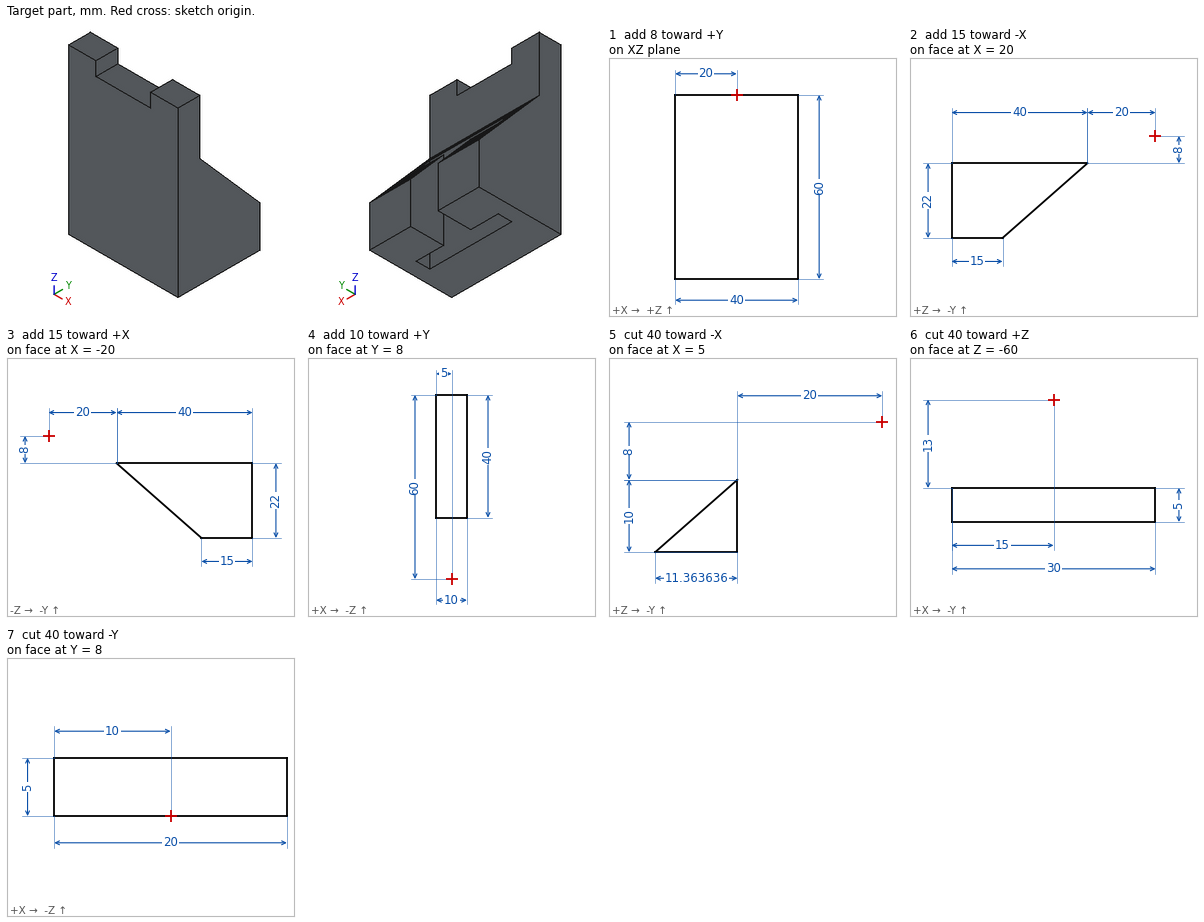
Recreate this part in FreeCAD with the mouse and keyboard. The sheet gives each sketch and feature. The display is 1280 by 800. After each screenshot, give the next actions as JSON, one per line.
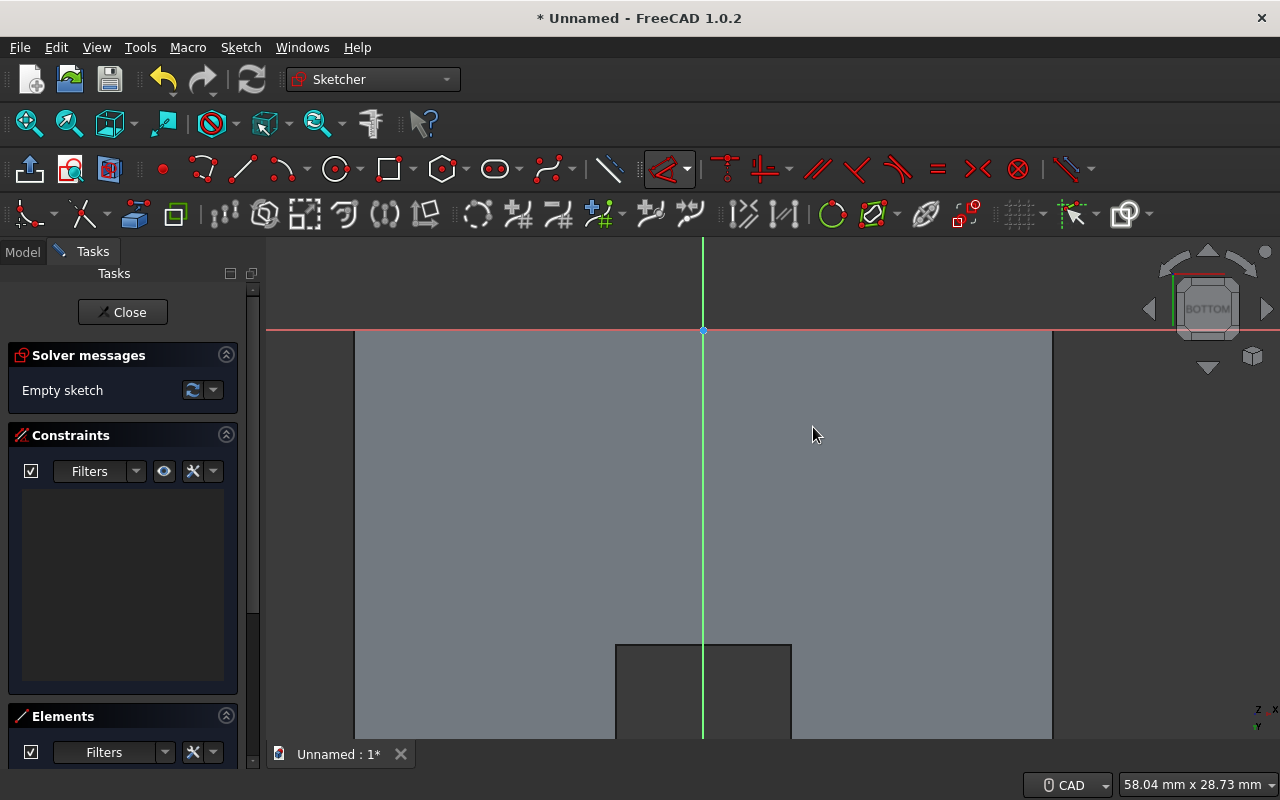
{"action": "left_click", "coordinate": [390, 170]}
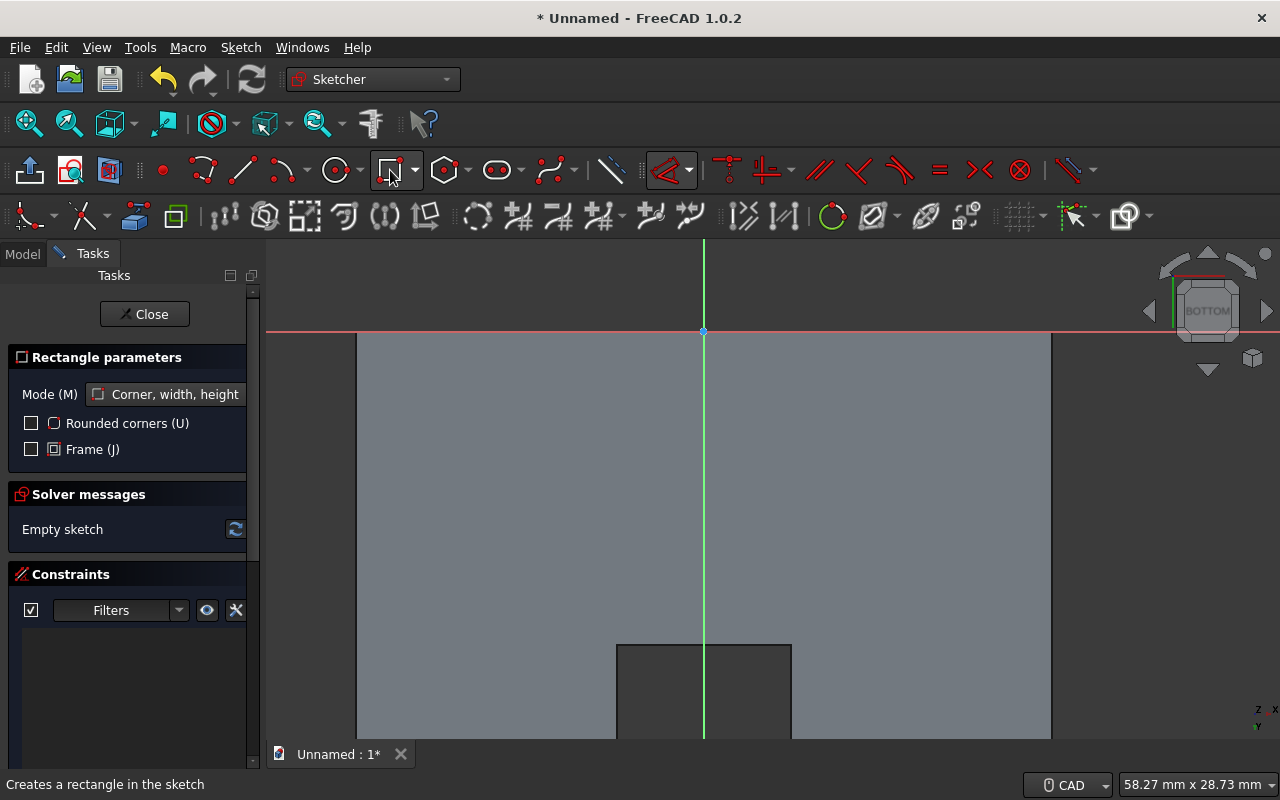
{"action": "left_click", "coordinate": [443, 558]}
{"action": "mouse_move", "coordinate": [965, 645]}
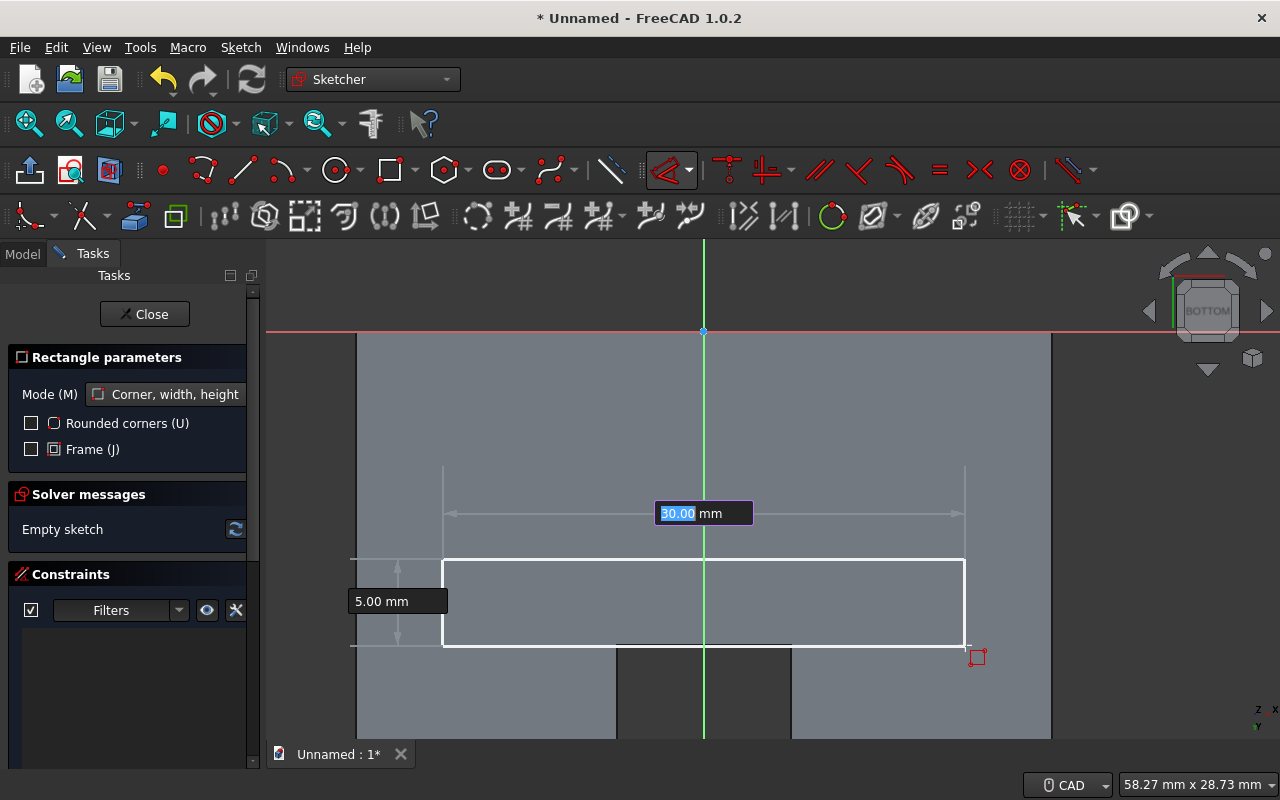
{"action": "type", "text": "30"}
{"action": "key", "text": "Tab"}
{"action": "type", "text": "5"}
{"action": "key", "text": "Return"}
{"action": "key", "text": "Escape"}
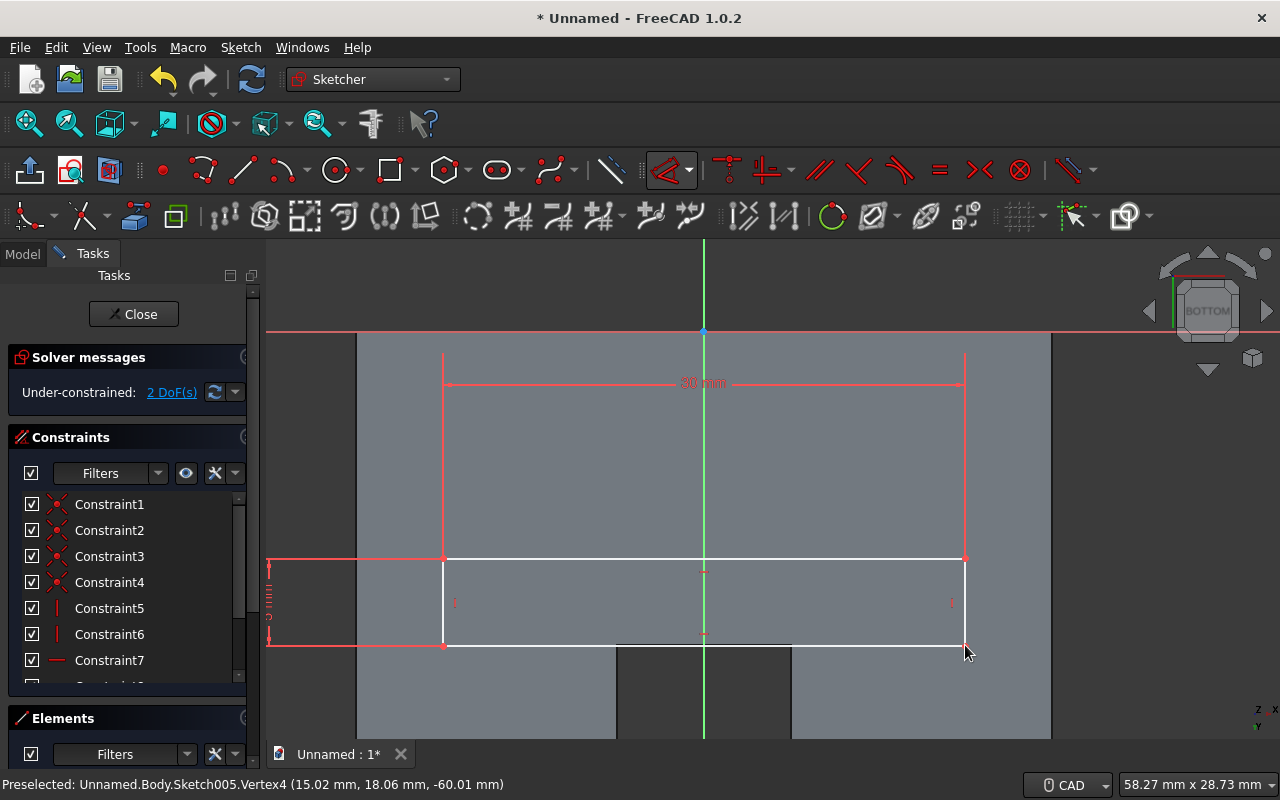
{"action": "left_click", "coordinate": [443, 559]}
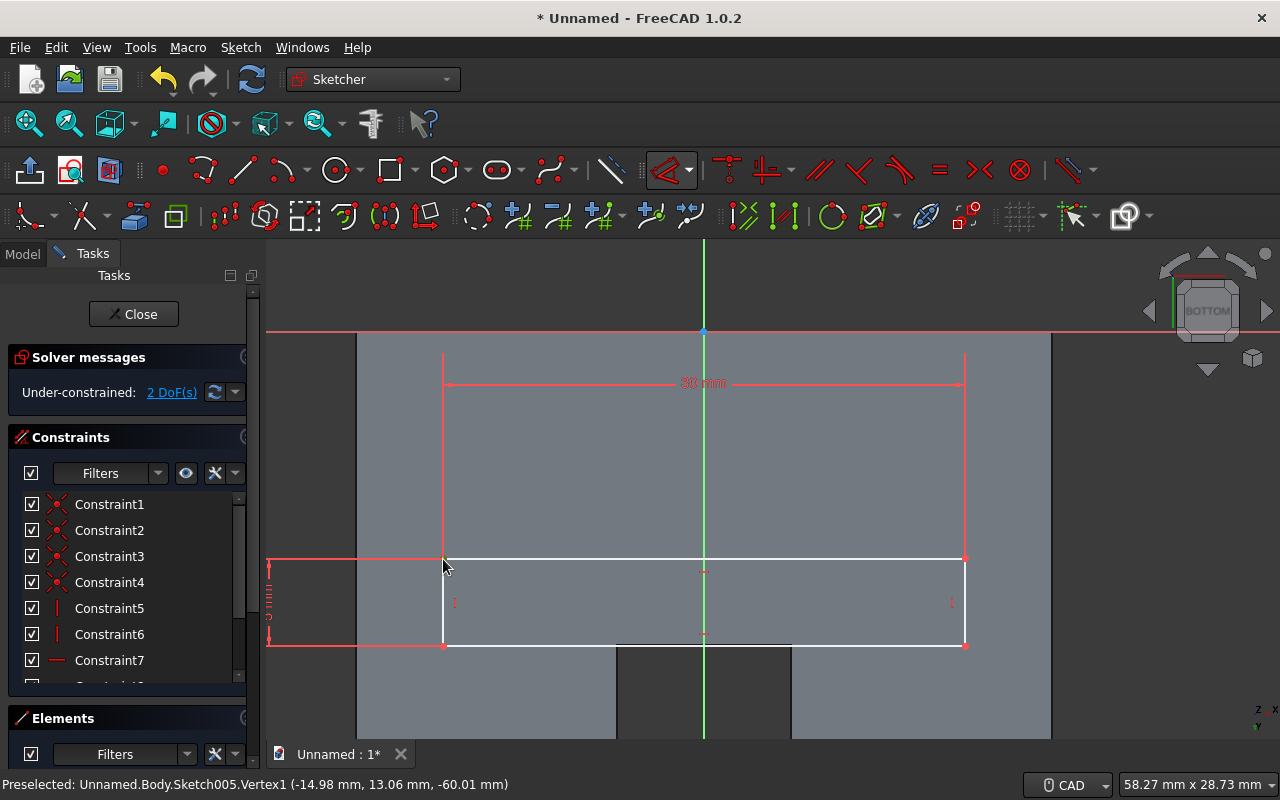
{"action": "key", "text": "l"}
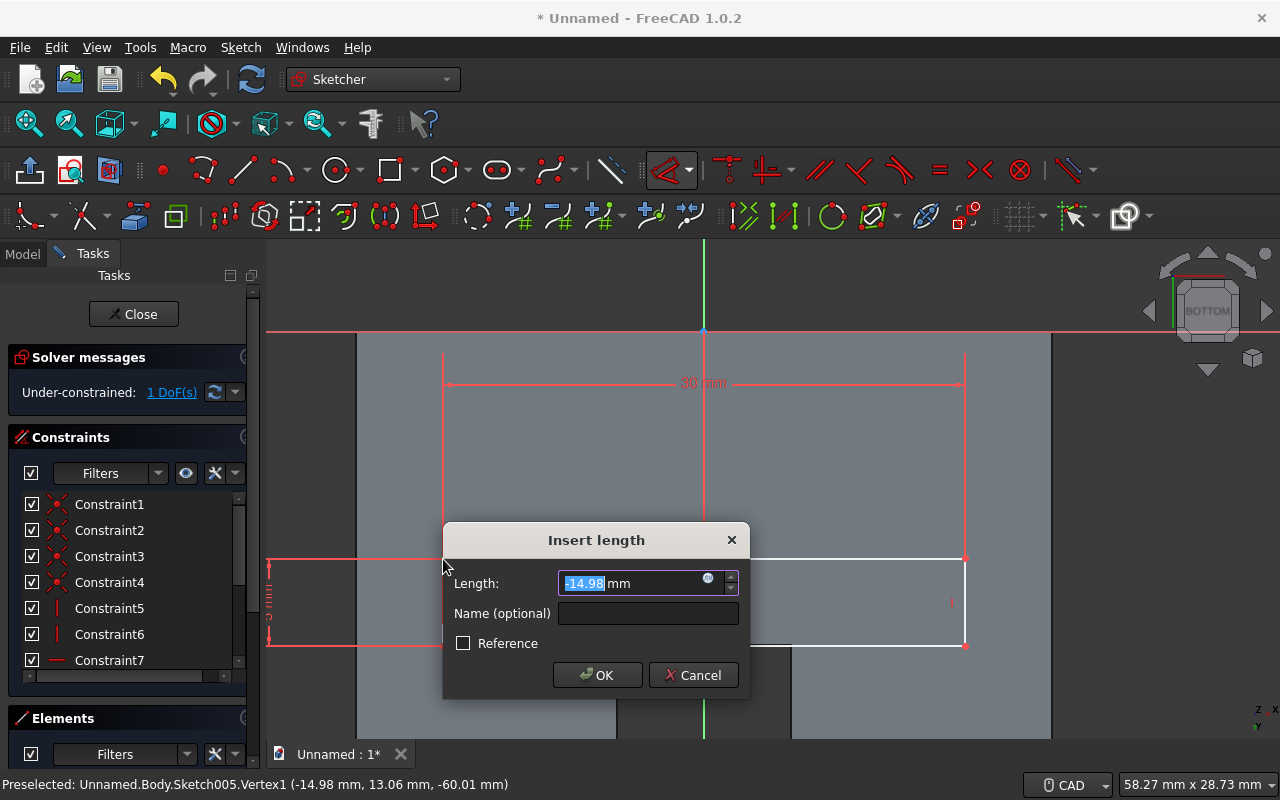
{"action": "type", "text": "-15"}
{"action": "key", "text": "Return"}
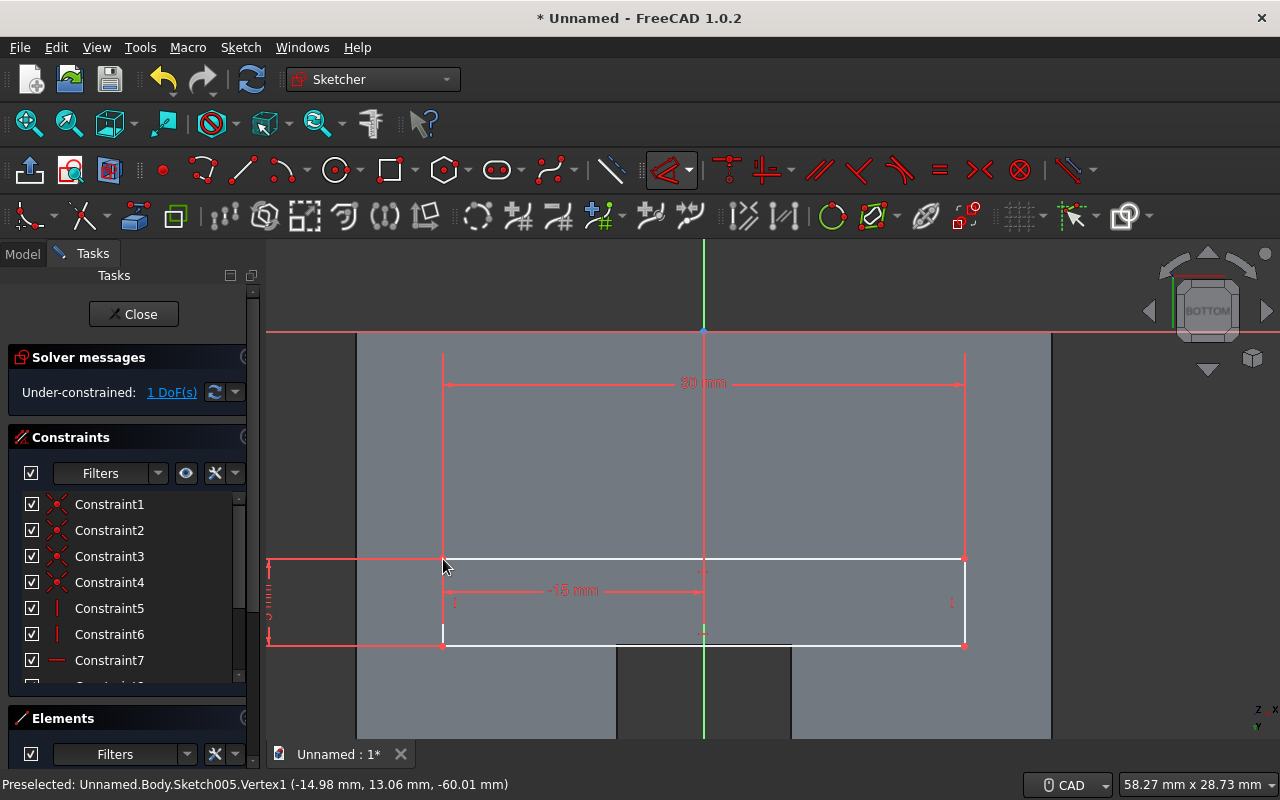
{"action": "left_click", "coordinate": [443, 559]}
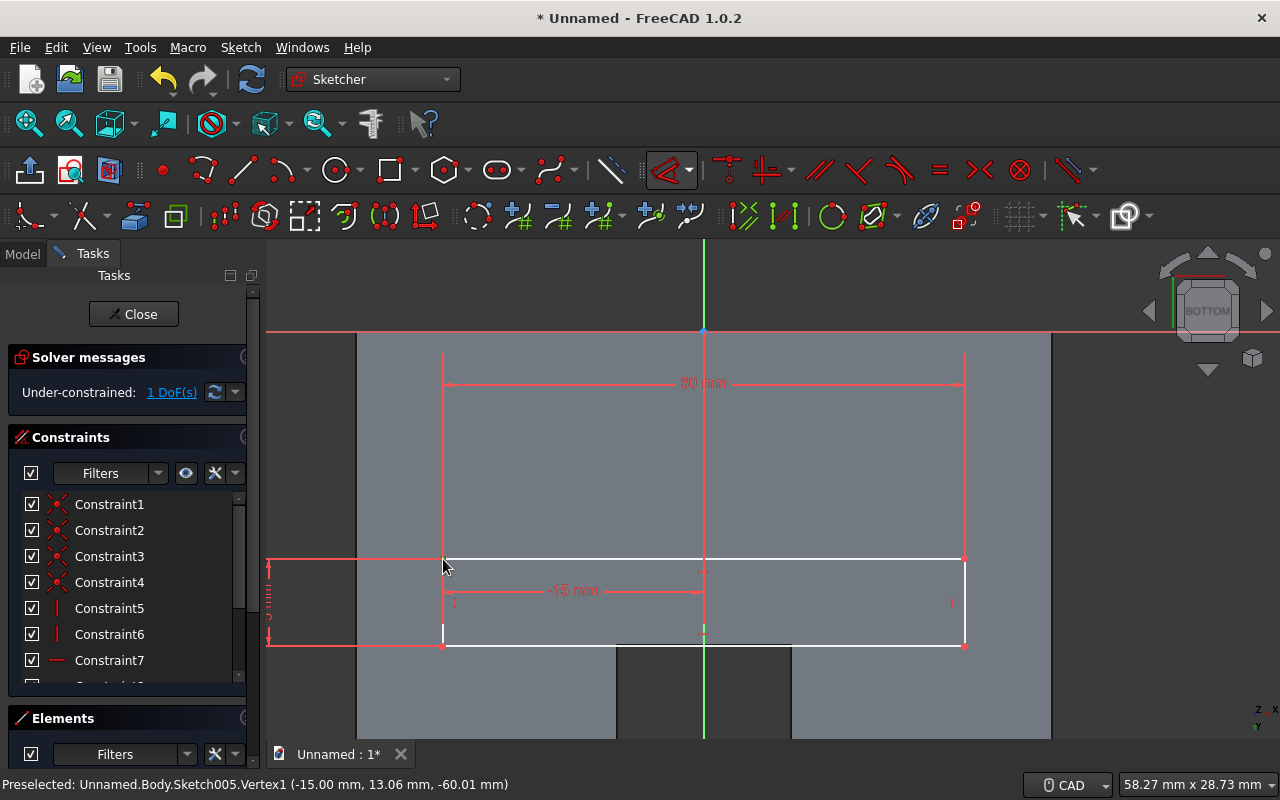
{"action": "key", "text": "i"}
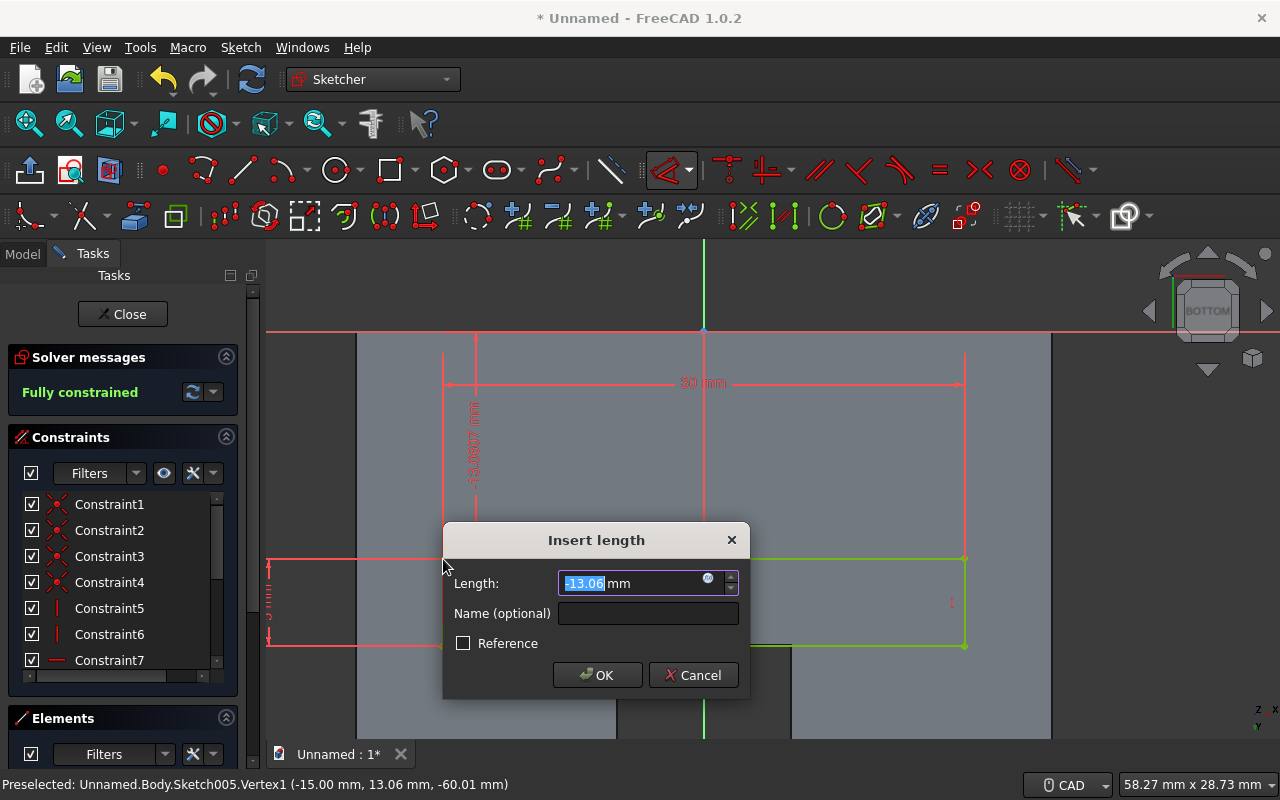
{"action": "type", "text": "-13"}
{"action": "key", "text": "Return"}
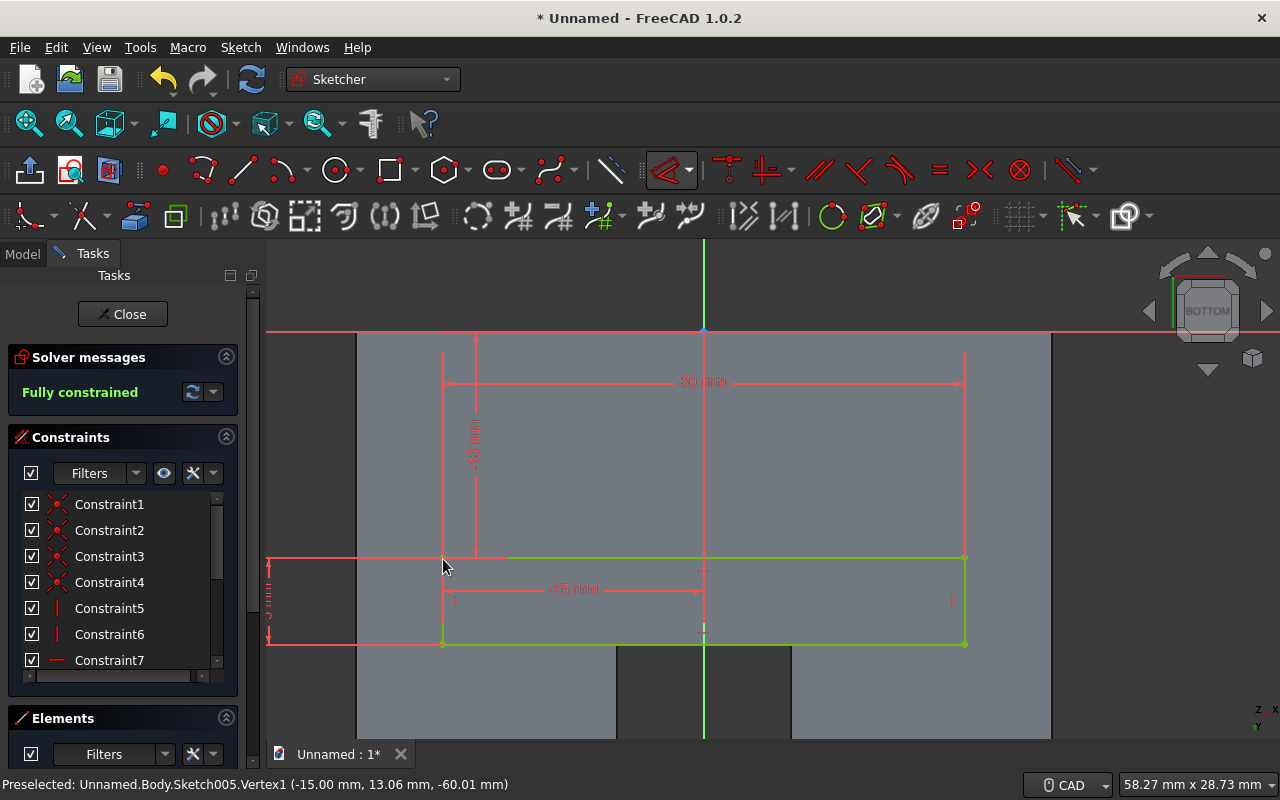
{"action": "left_click", "coordinate": [123, 314]}